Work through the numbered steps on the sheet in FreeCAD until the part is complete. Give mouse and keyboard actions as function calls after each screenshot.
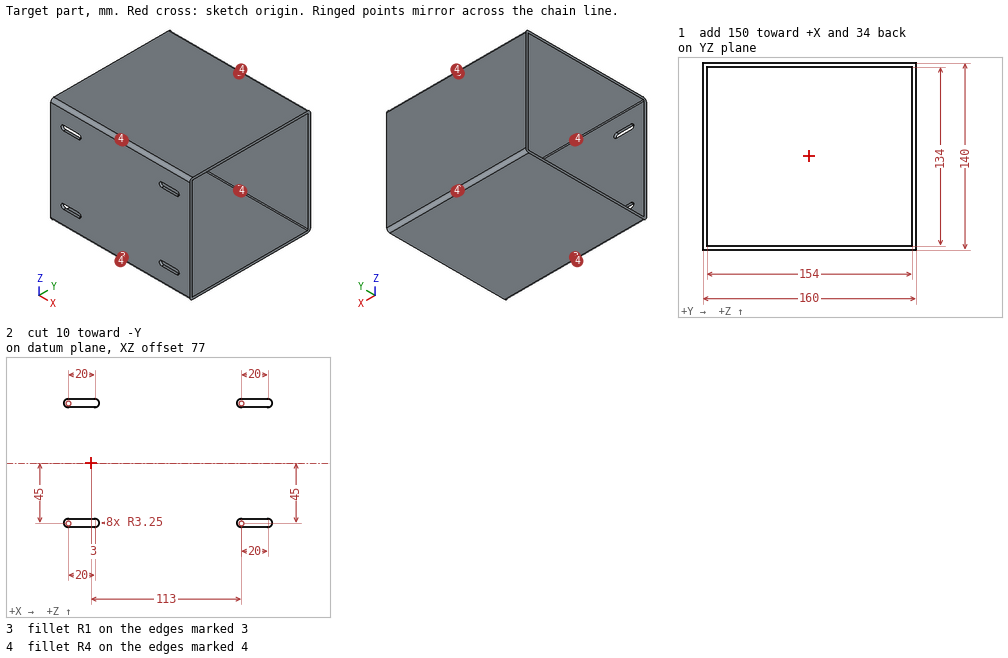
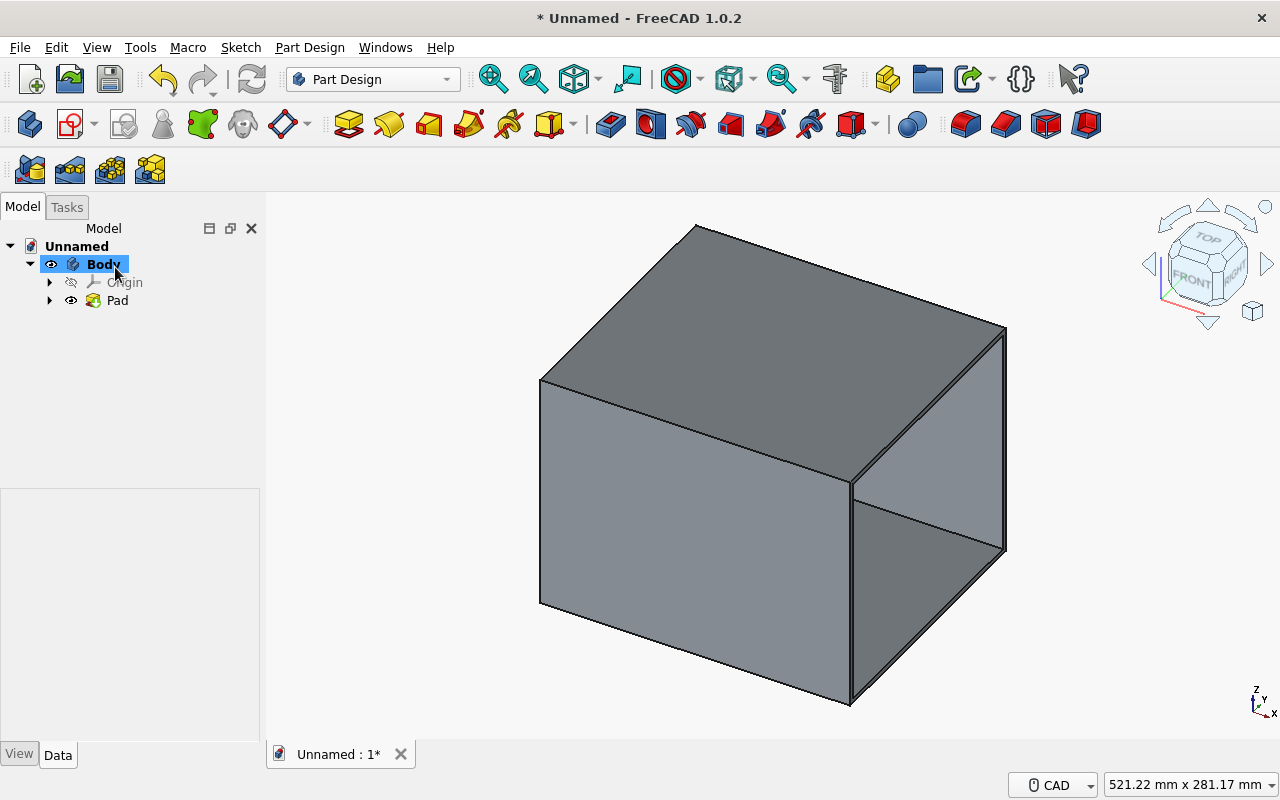
click(50, 282)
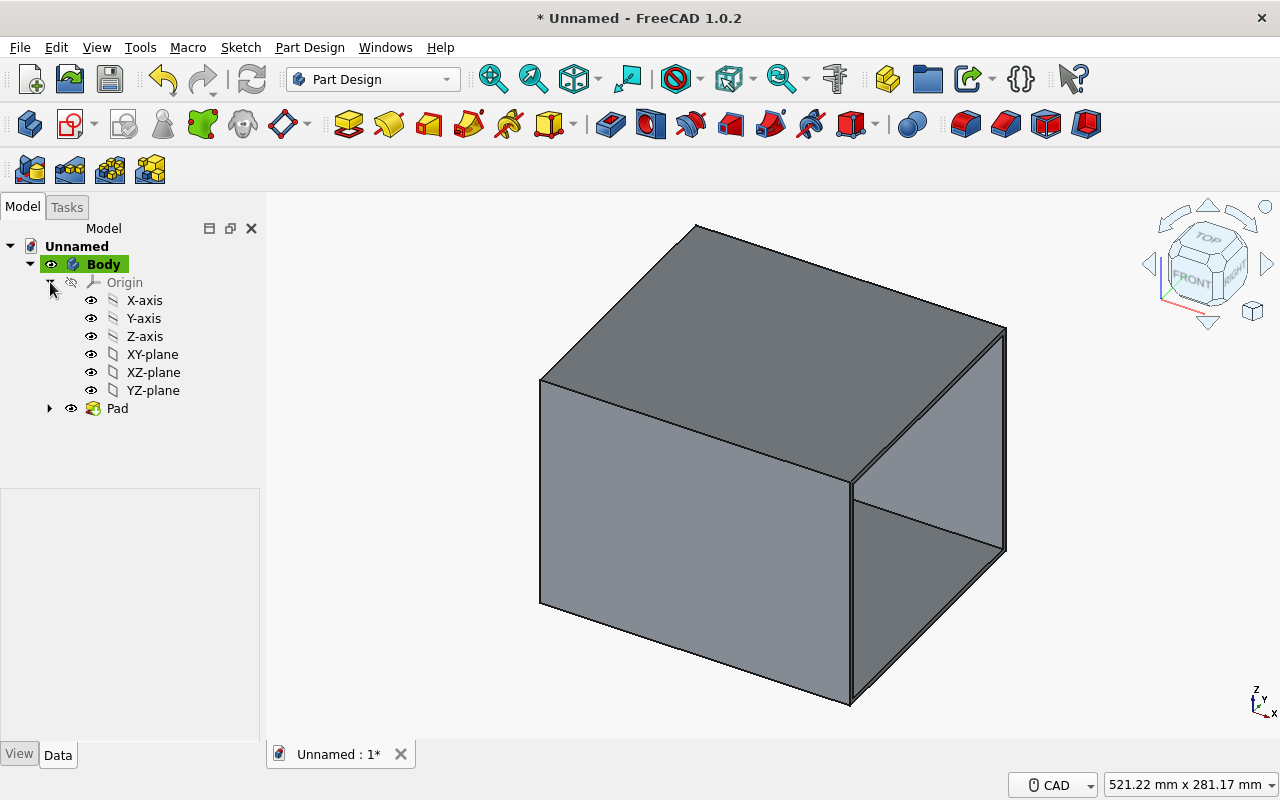
click(136, 372)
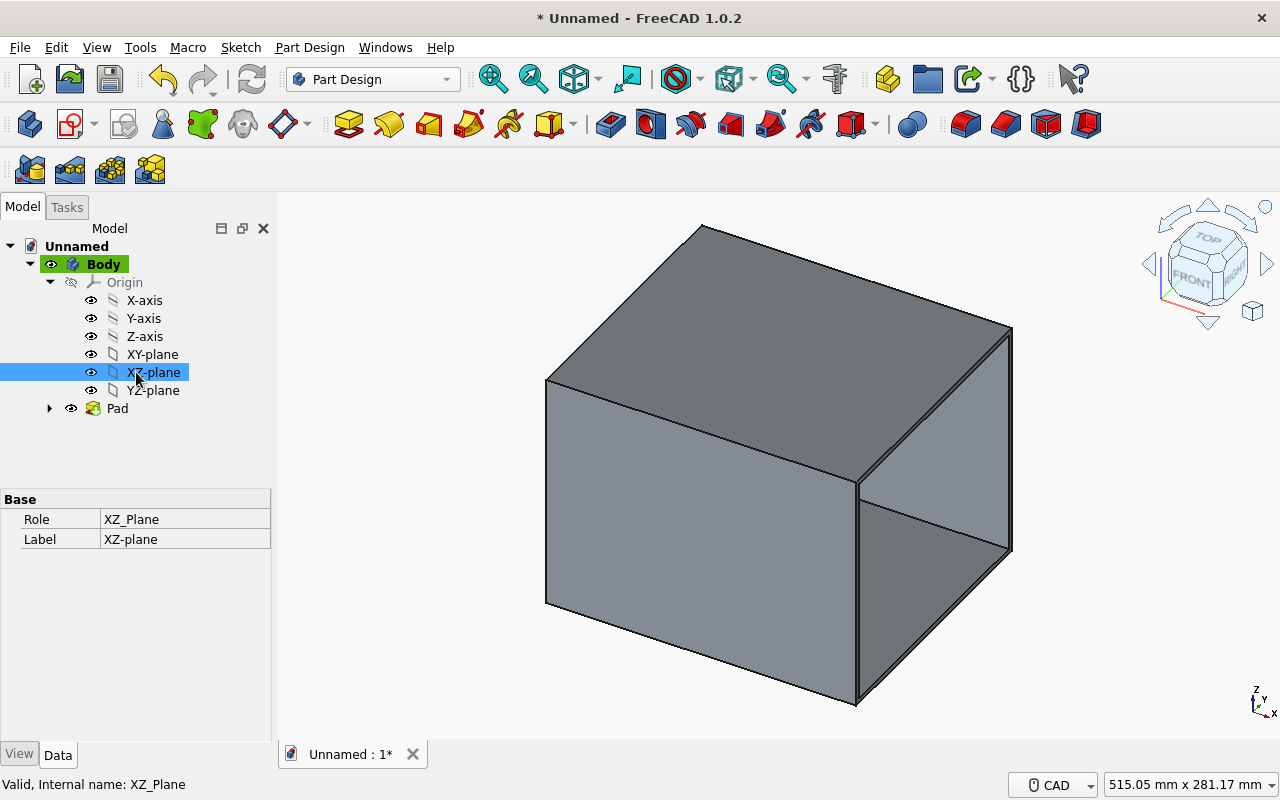
click(284, 124)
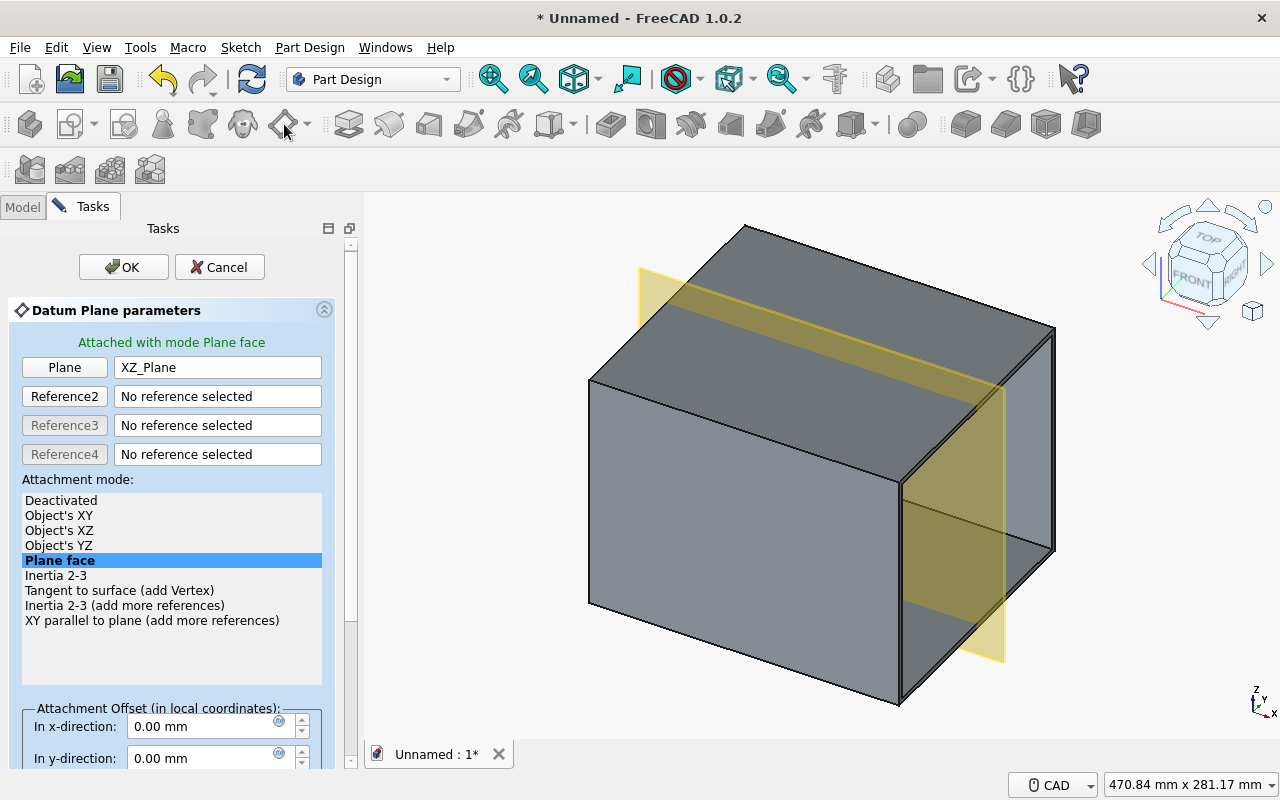
scroll(351, 503, down, 2)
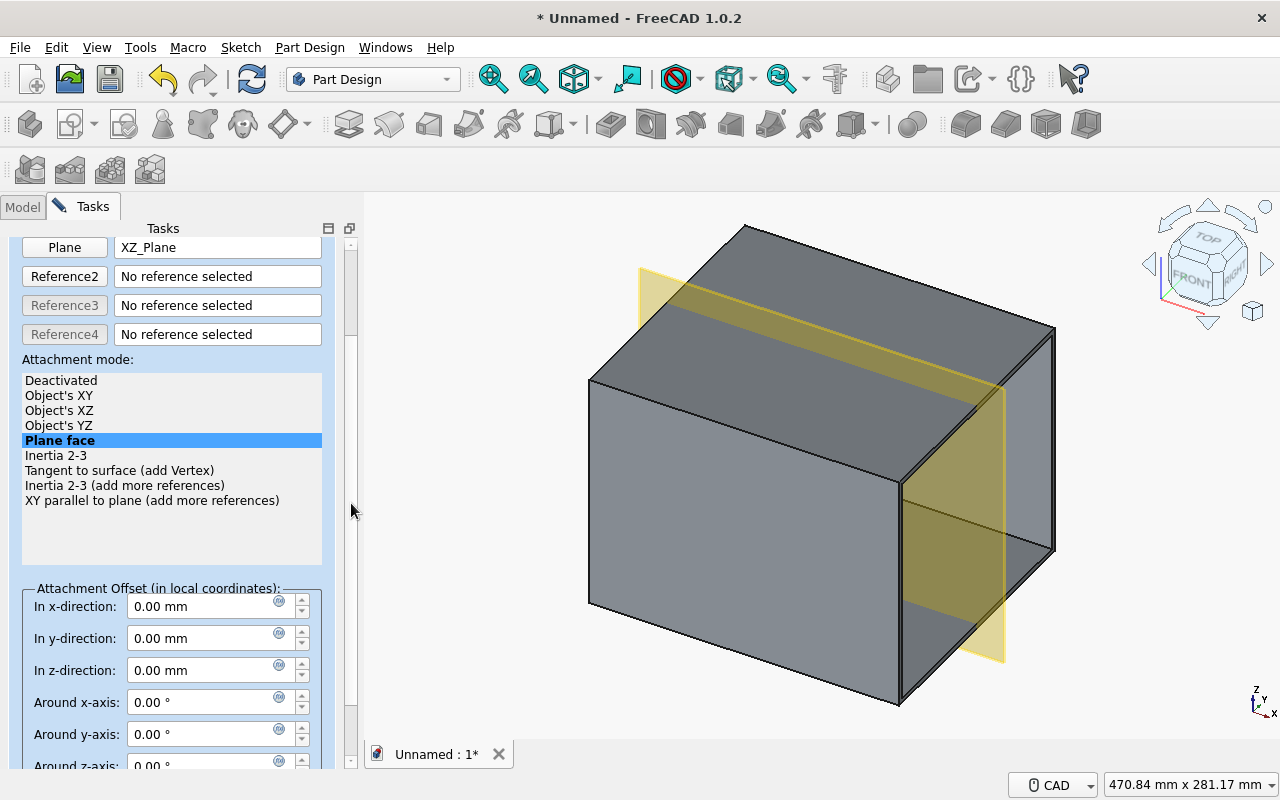
triple_click(210, 670)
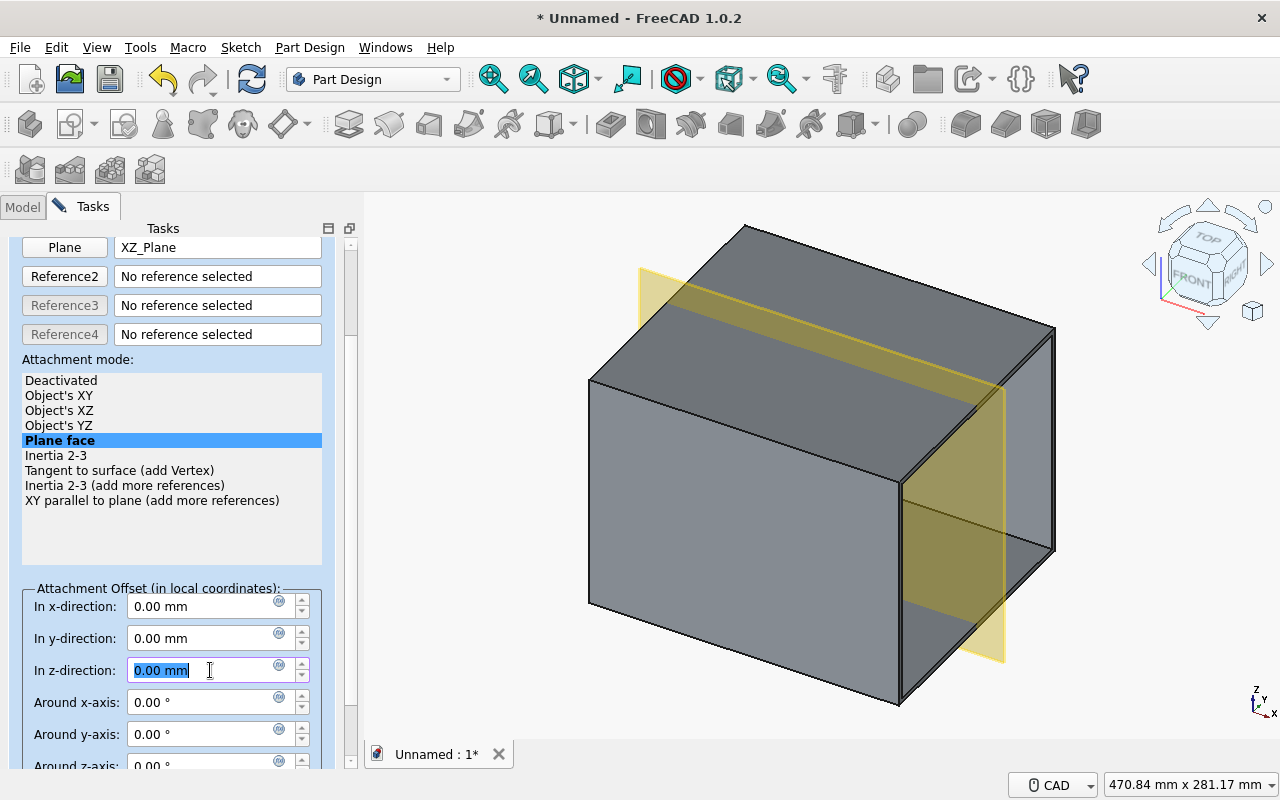
text(77)
key(Tab)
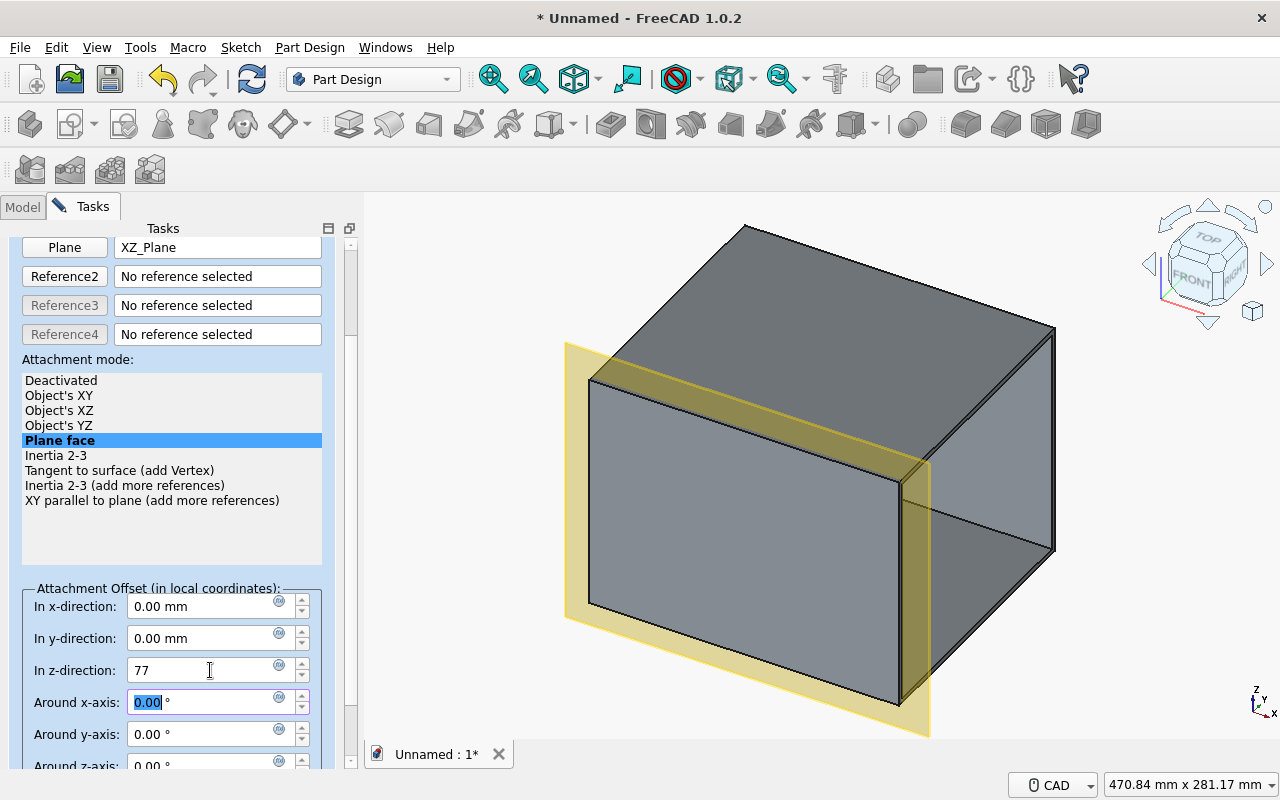
scroll(351, 503, up, 3)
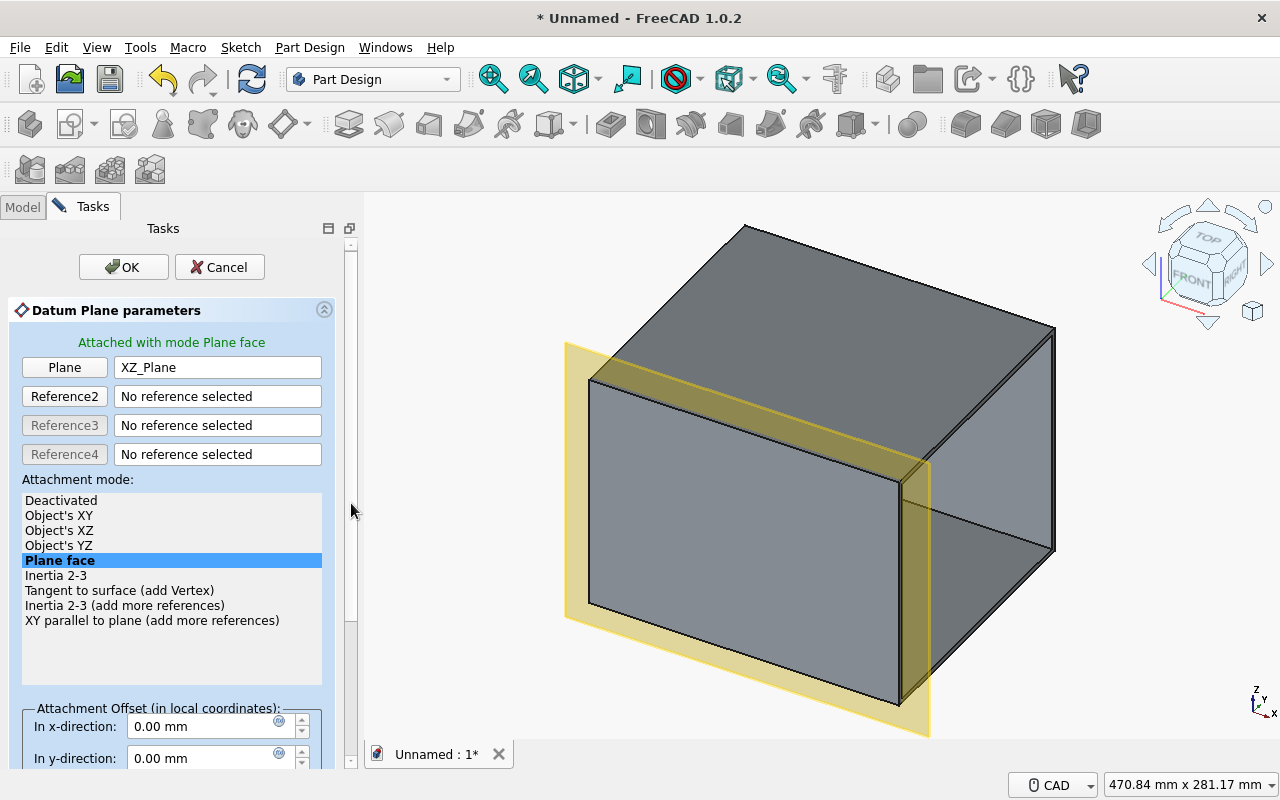
click(124, 267)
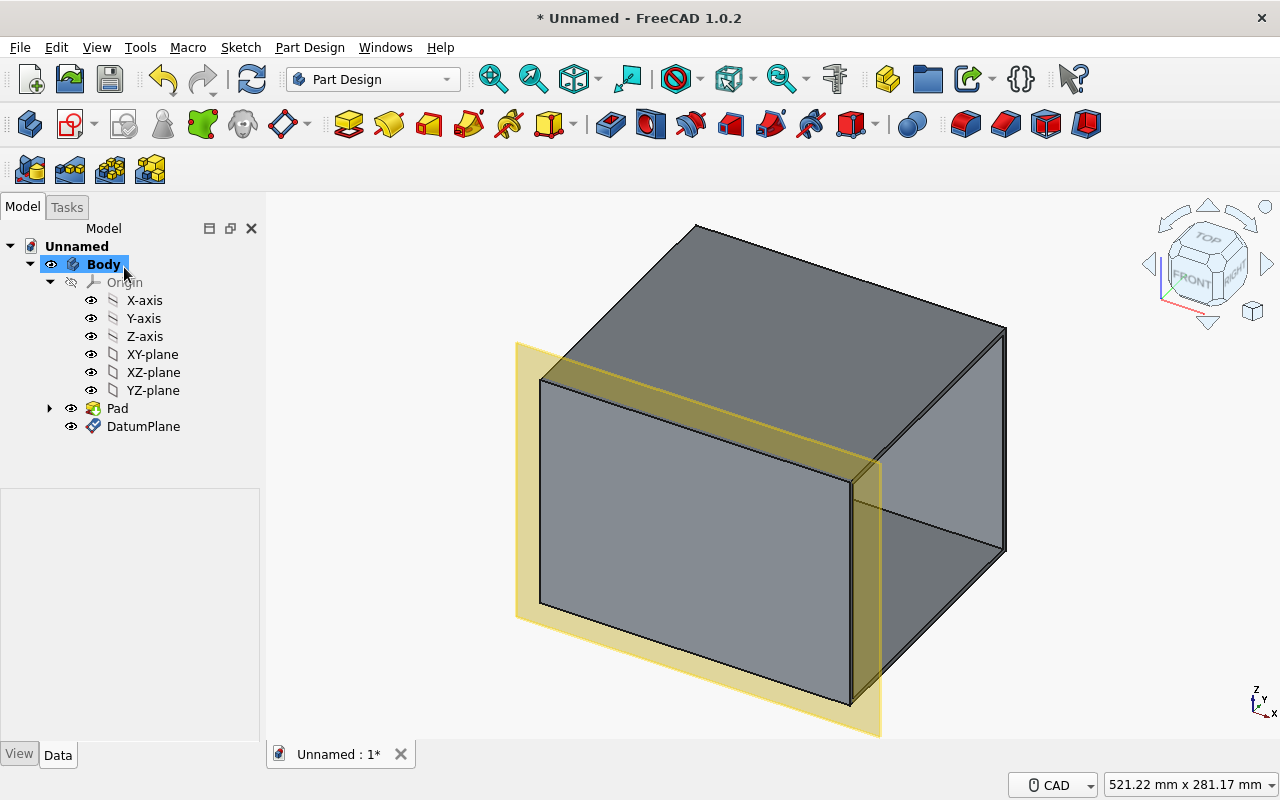
click(116, 426)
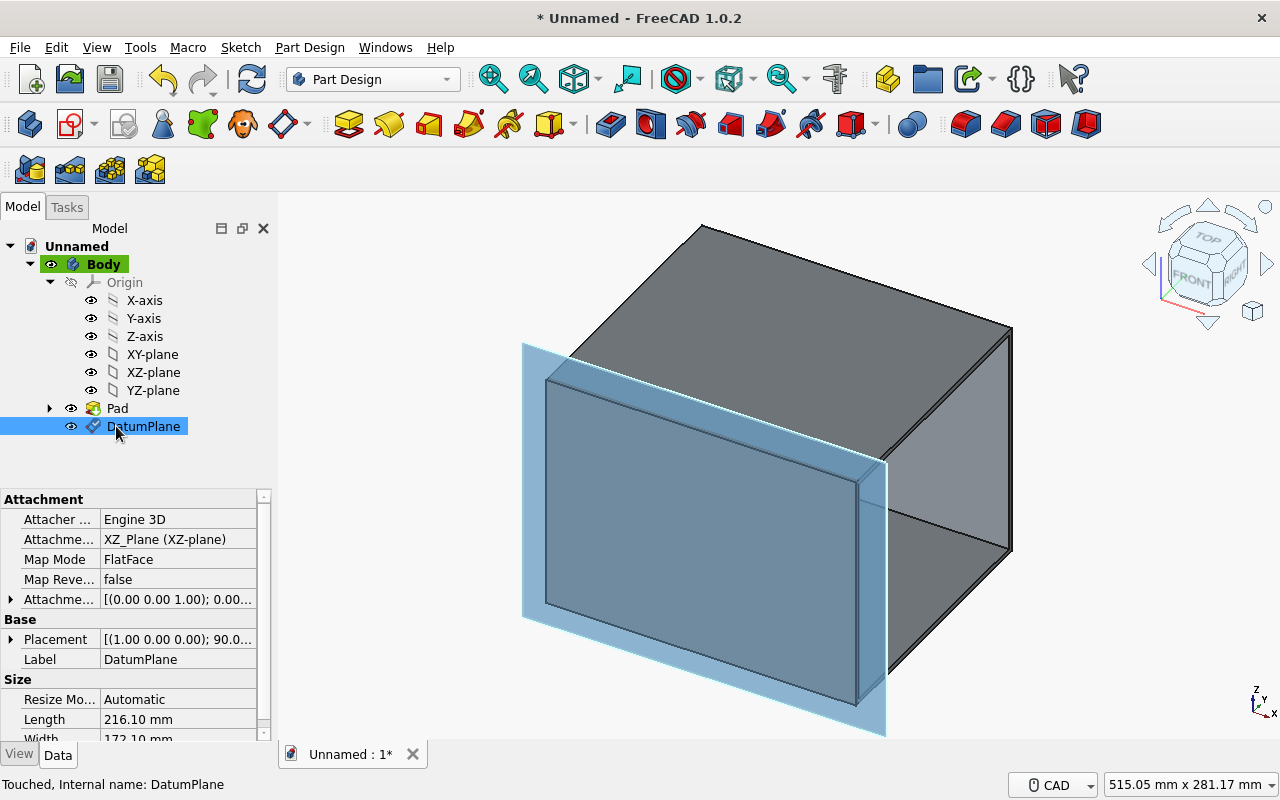
click(70, 124)